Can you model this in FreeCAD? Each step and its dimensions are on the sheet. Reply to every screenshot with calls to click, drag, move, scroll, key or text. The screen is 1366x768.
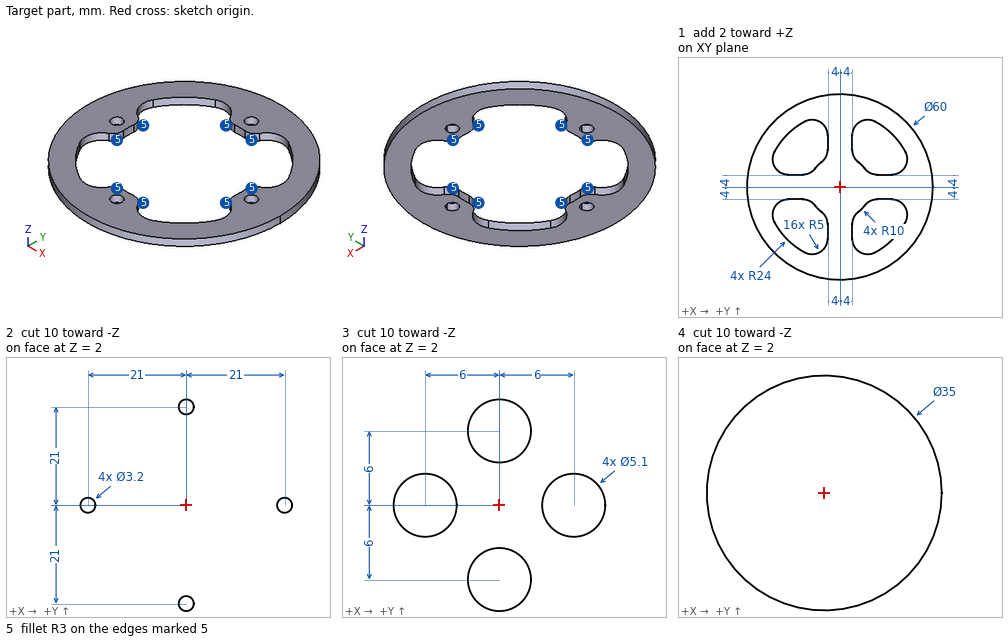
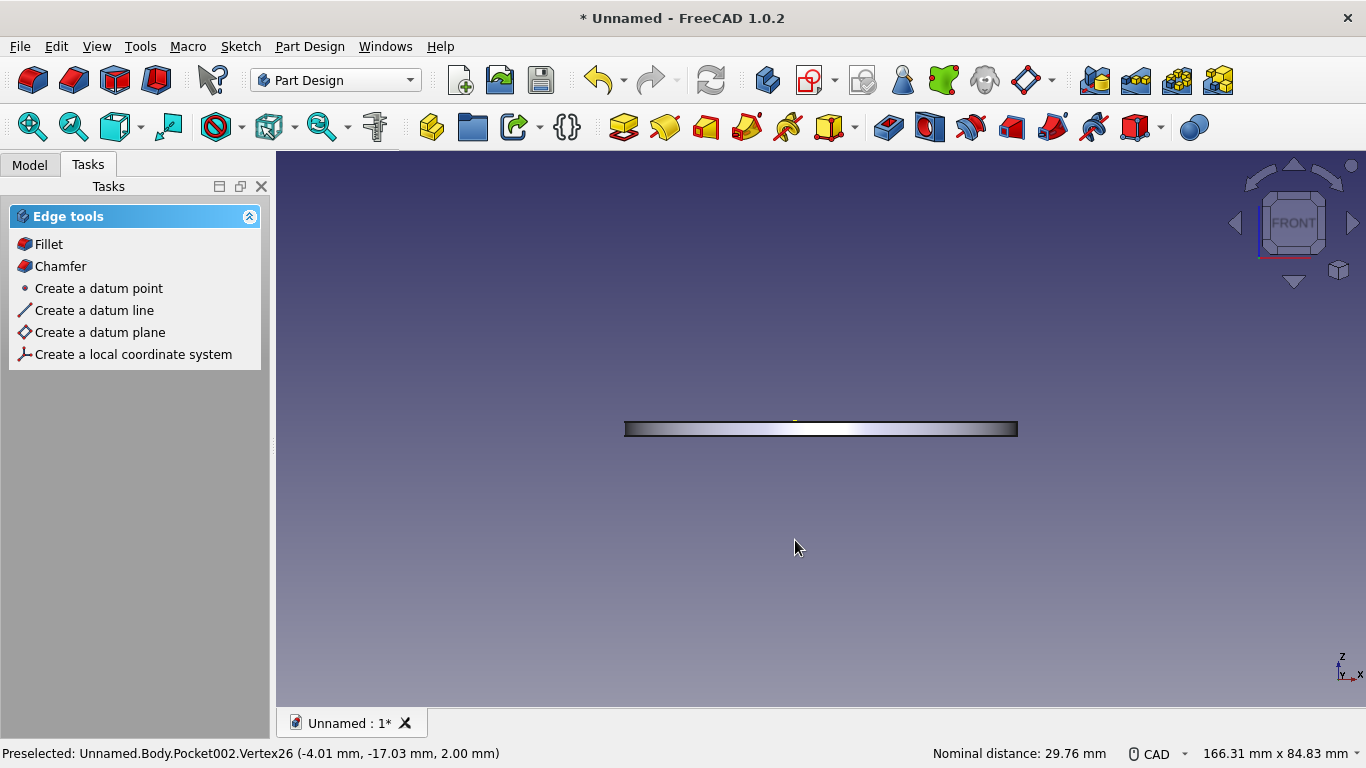
key(v)
key(f)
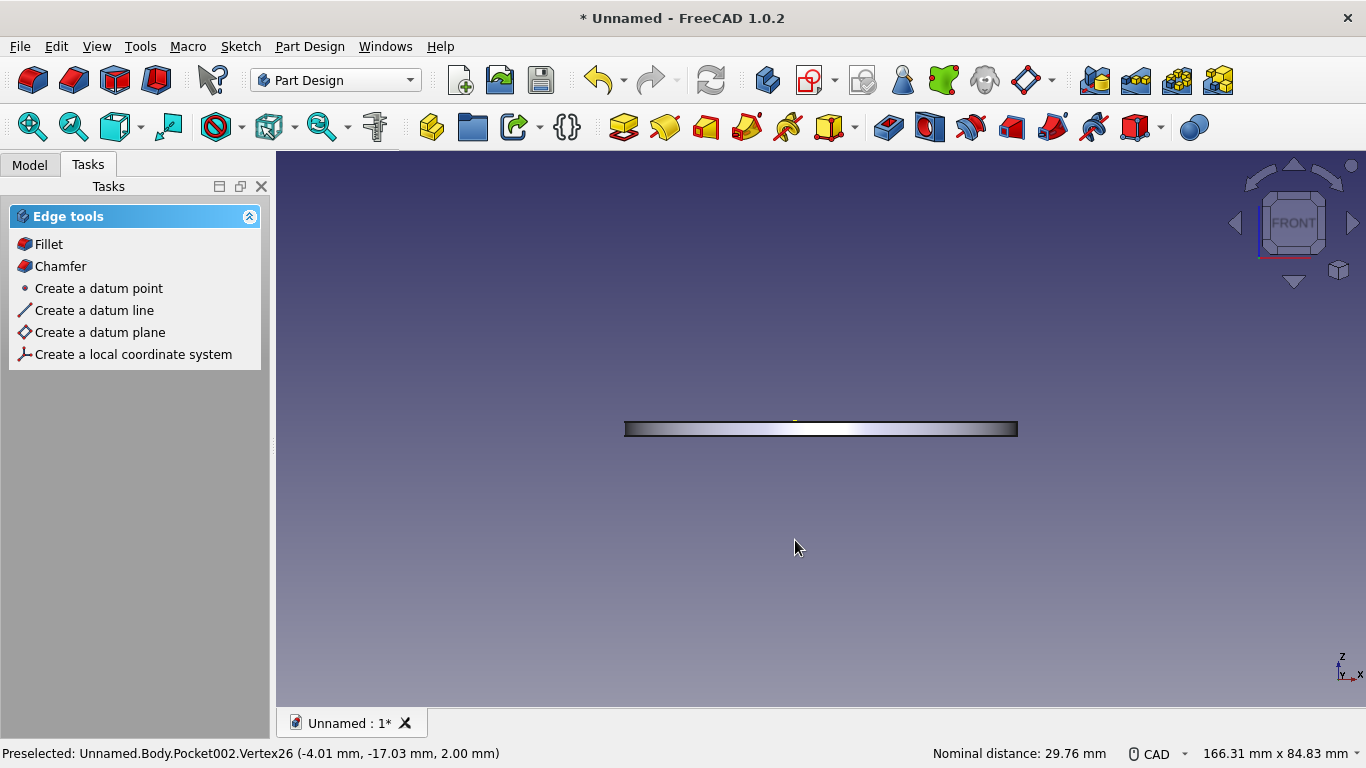
scroll(795, 428, up, 6)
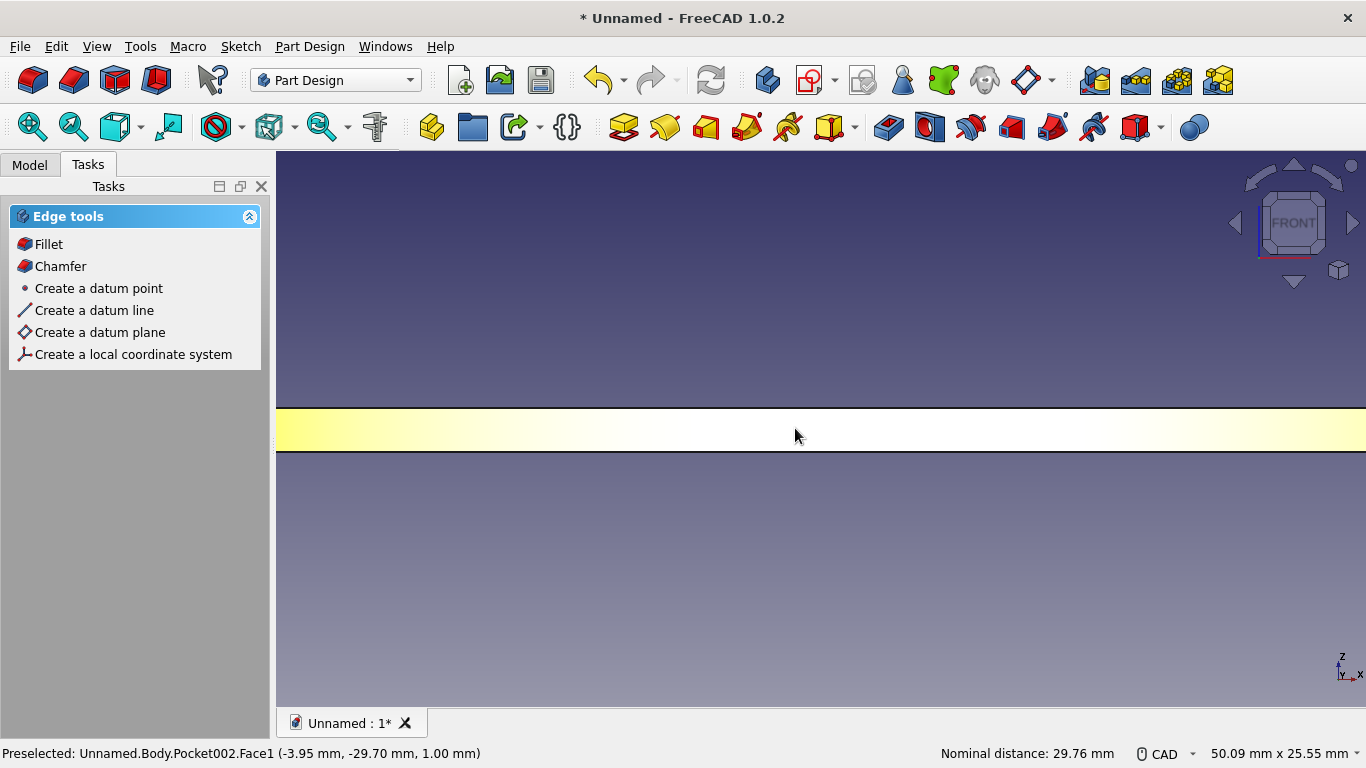
key(v)
key(f)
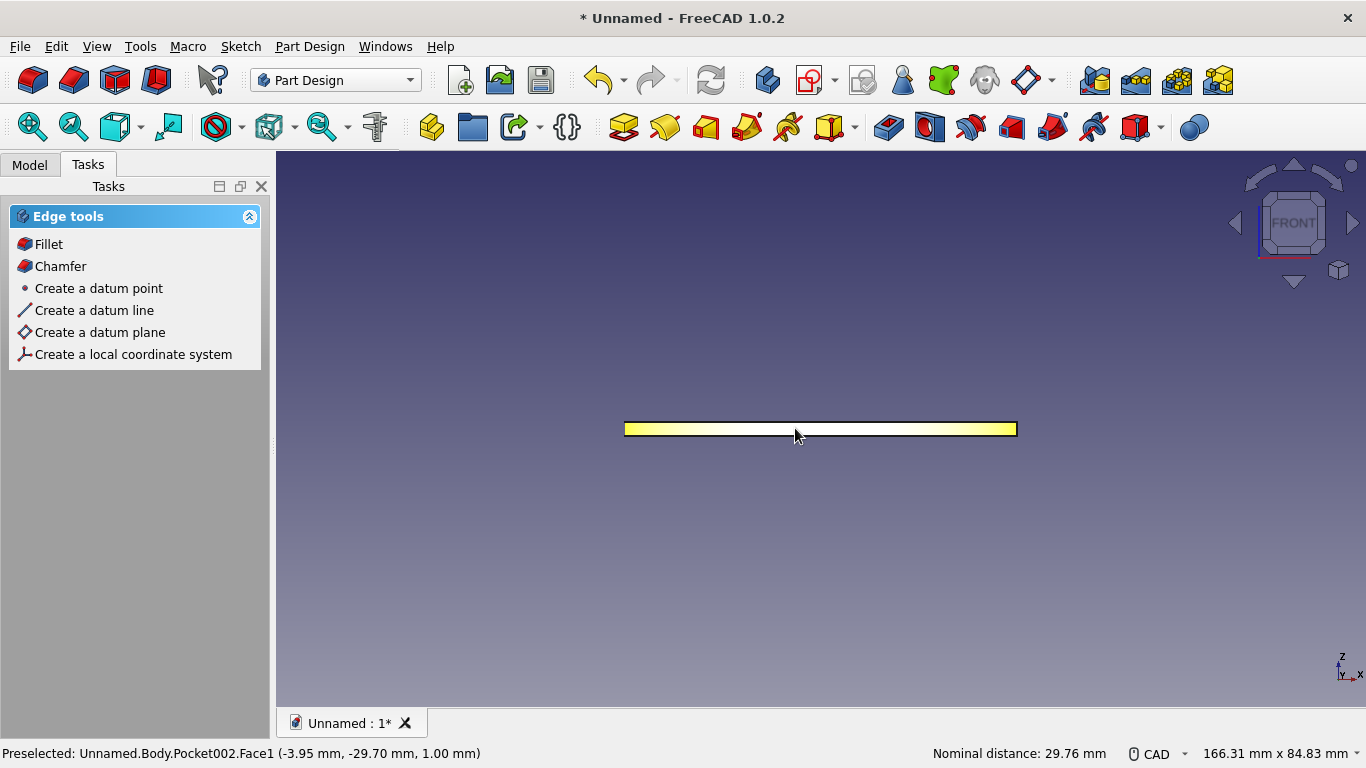
key(3)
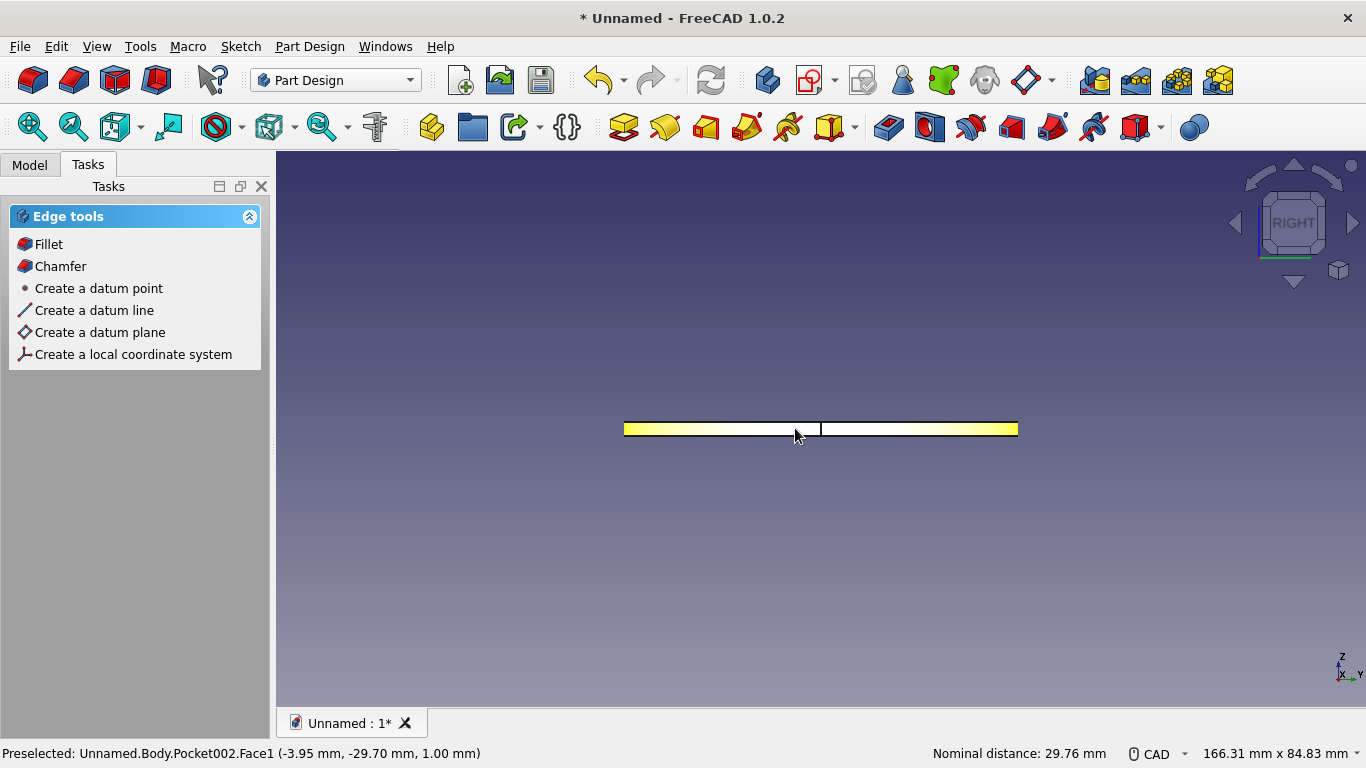
key(v)
key(f)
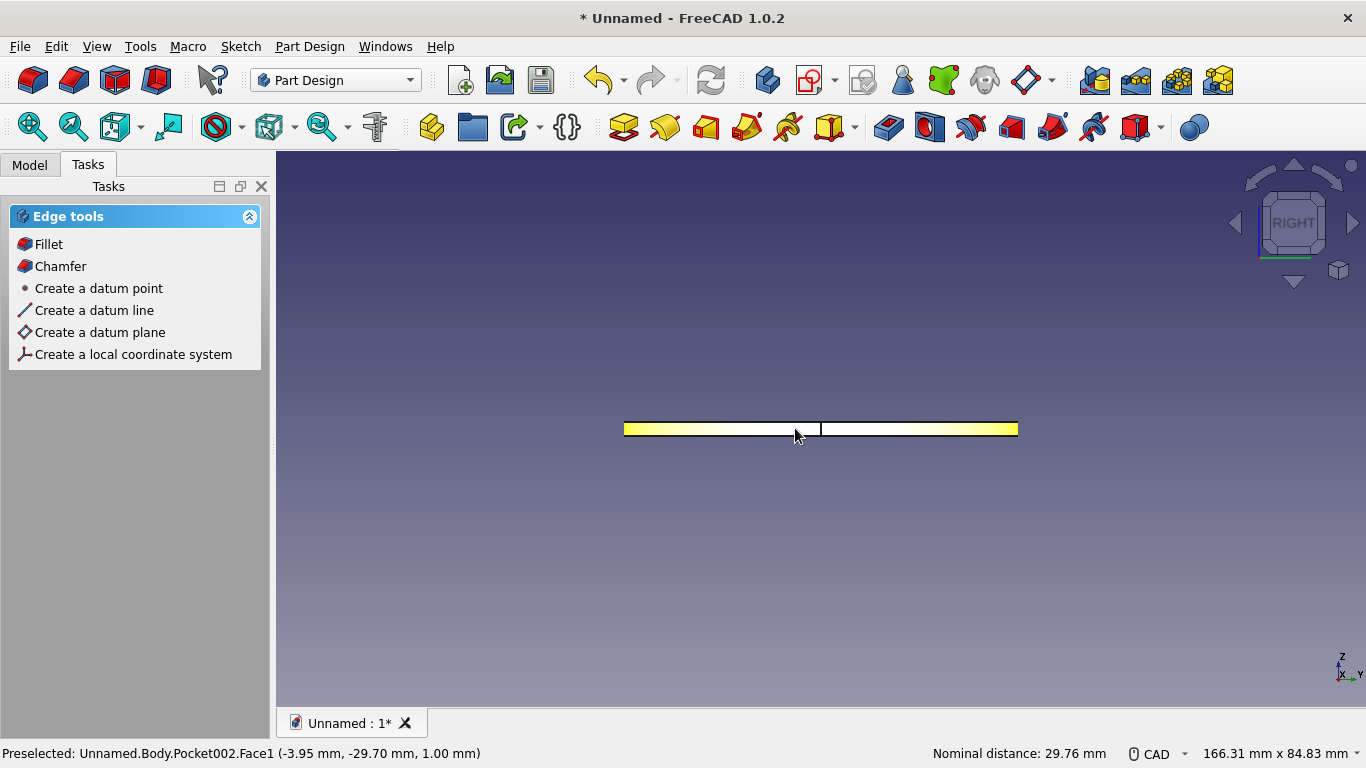
scroll(709, 428, up, 6)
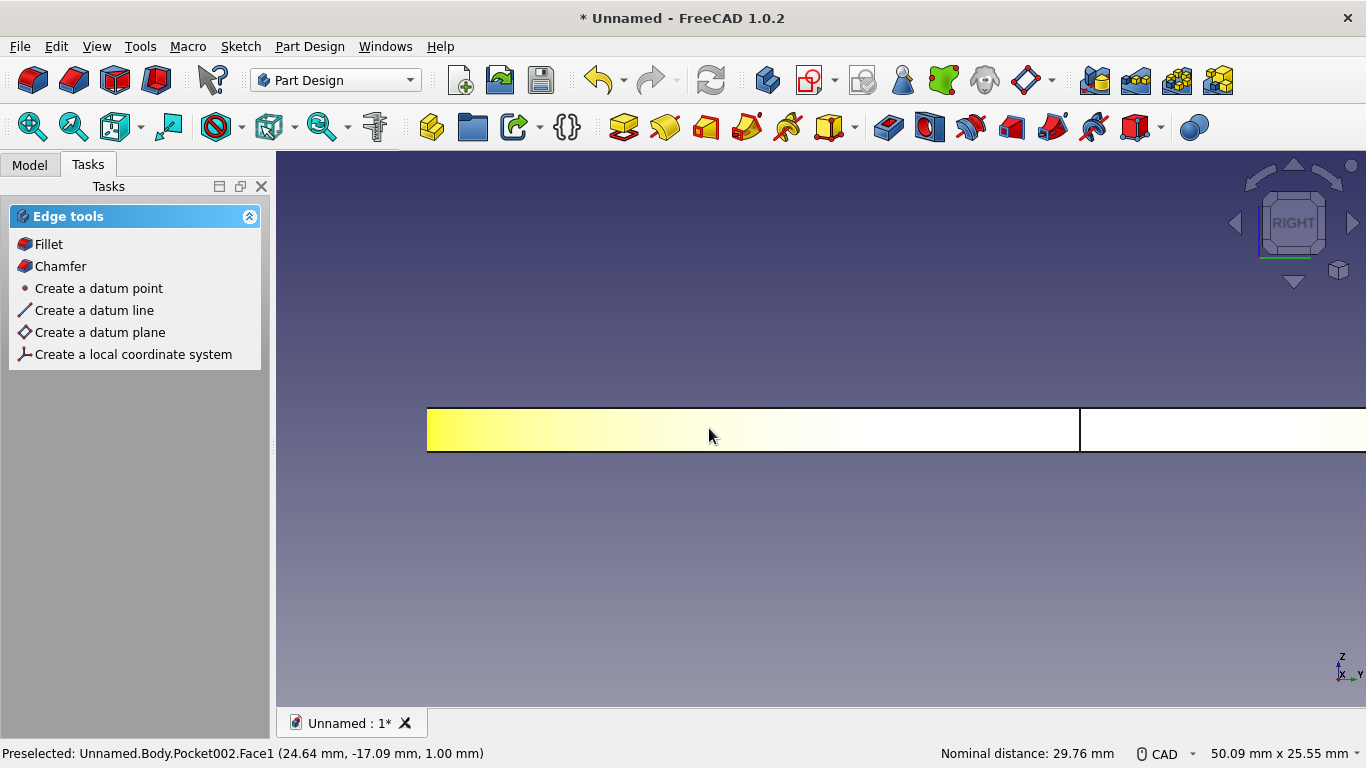
click(33, 128)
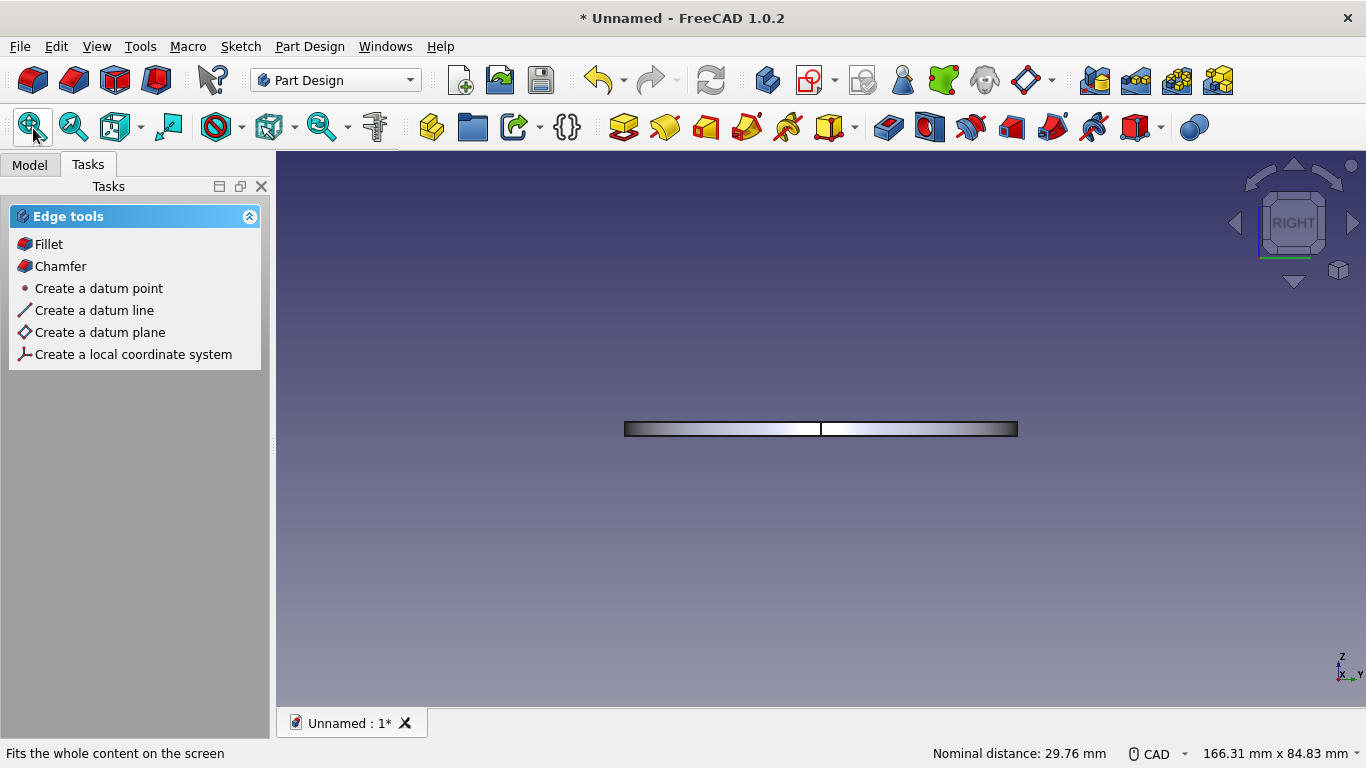
key(5)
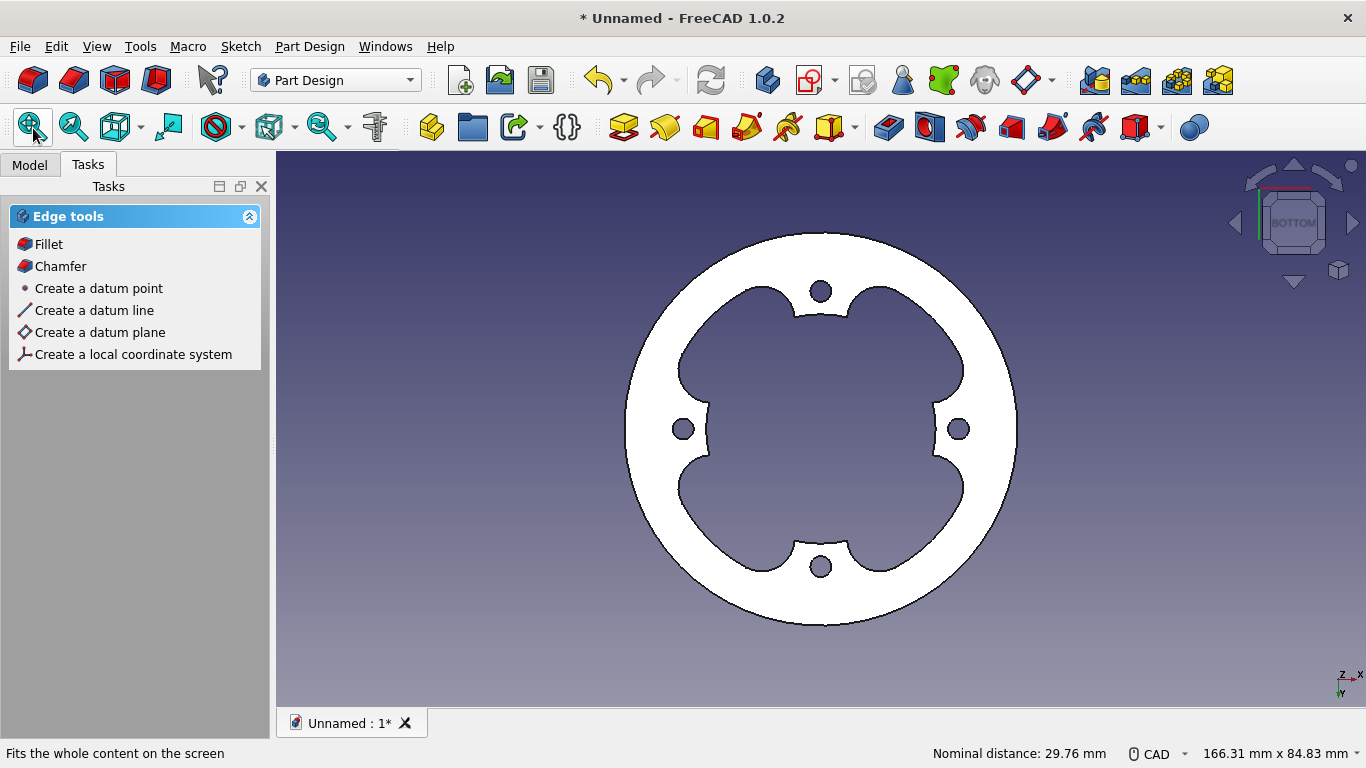
scroll(795, 316, up, 6)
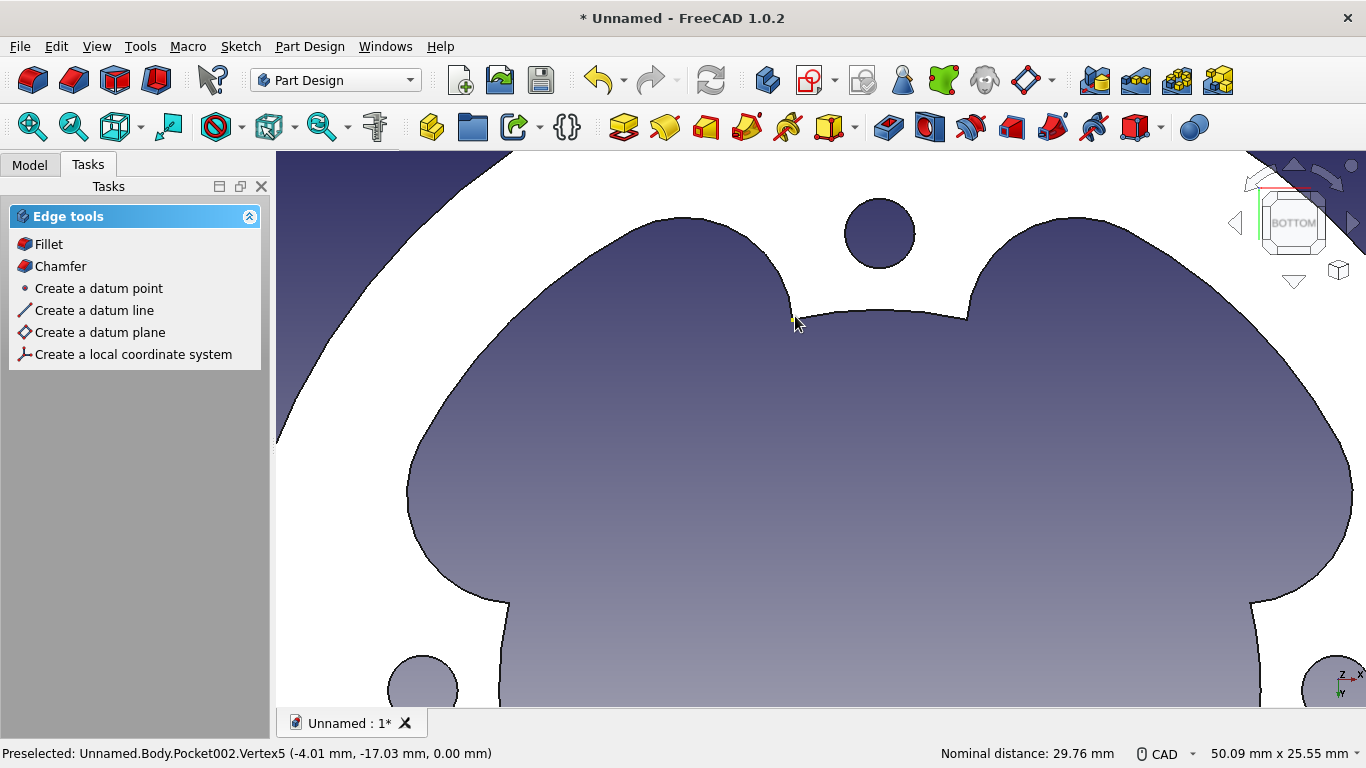
key(v)
key(f)